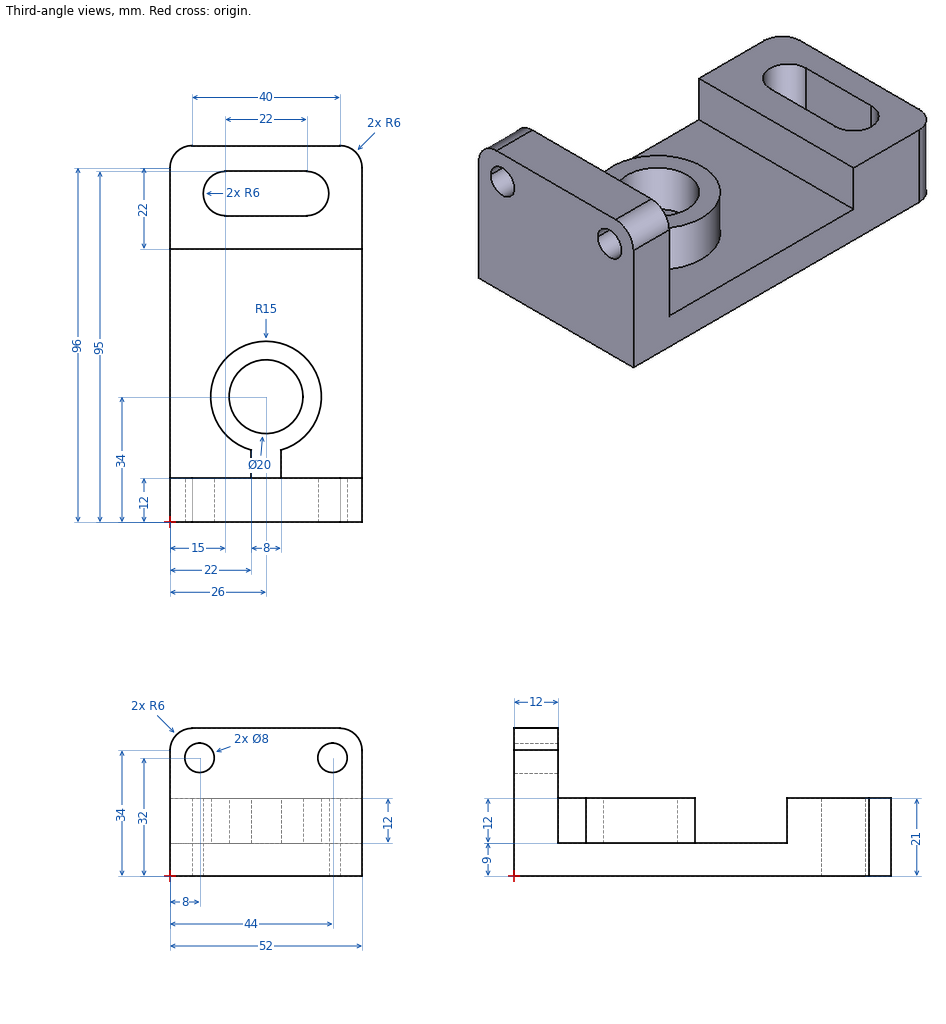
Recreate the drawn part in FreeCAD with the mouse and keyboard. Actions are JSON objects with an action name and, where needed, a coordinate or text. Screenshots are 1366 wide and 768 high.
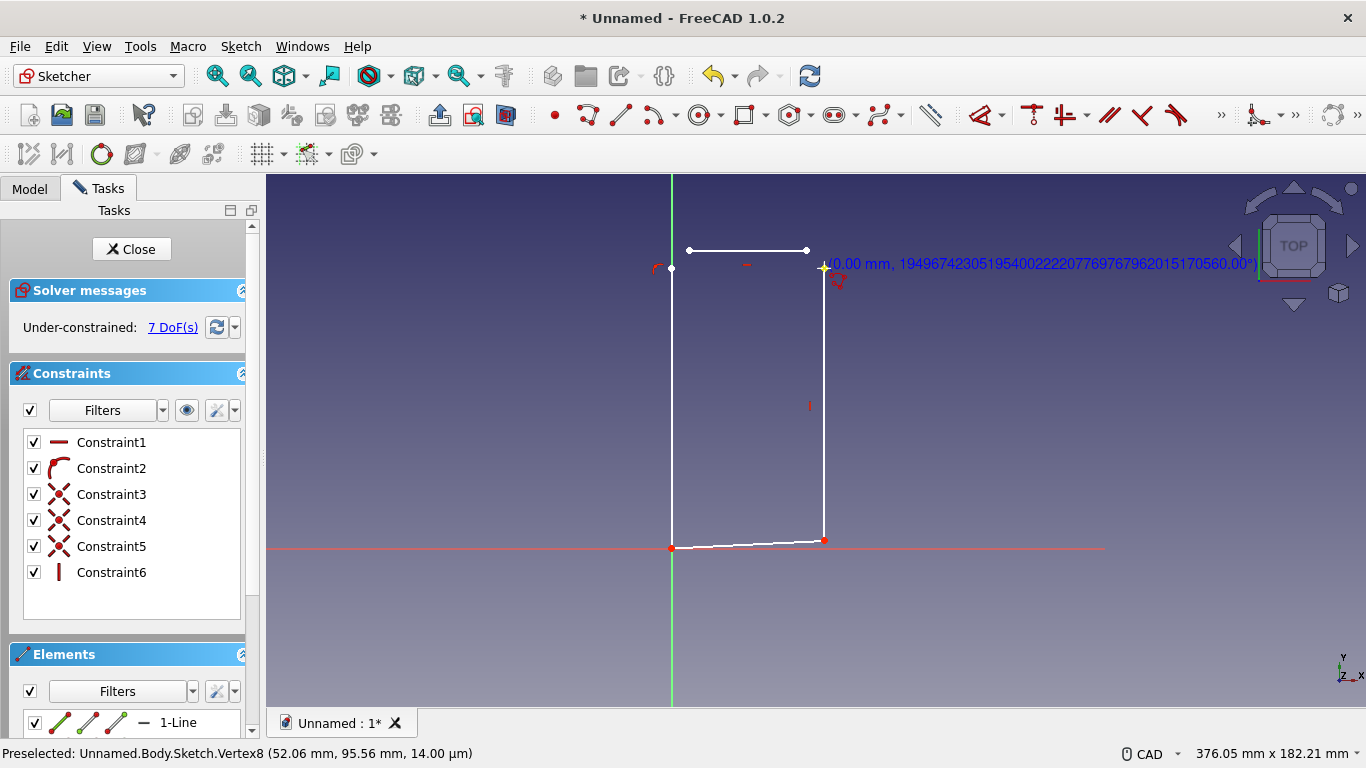
{"action": "left_click", "coordinate": [676, 116]}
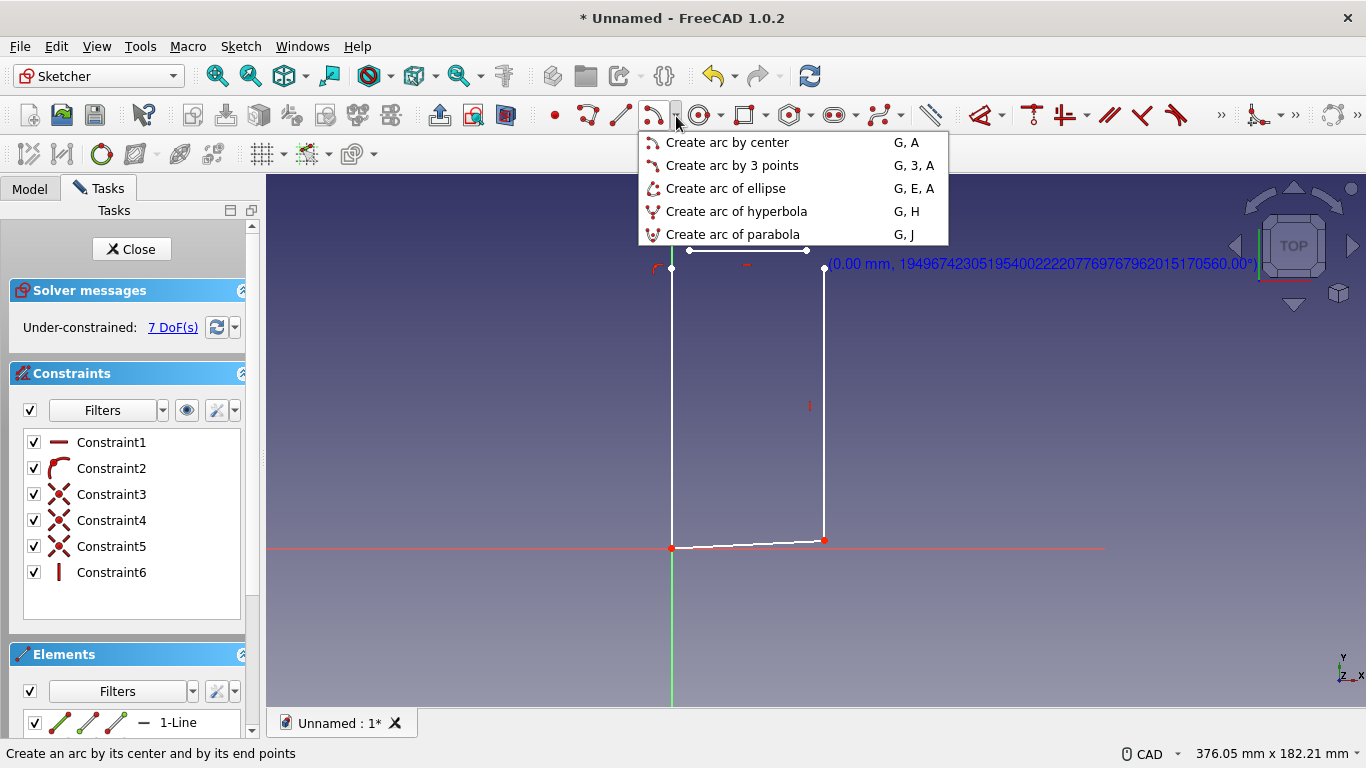
{"action": "left_click", "coordinate": [794, 166]}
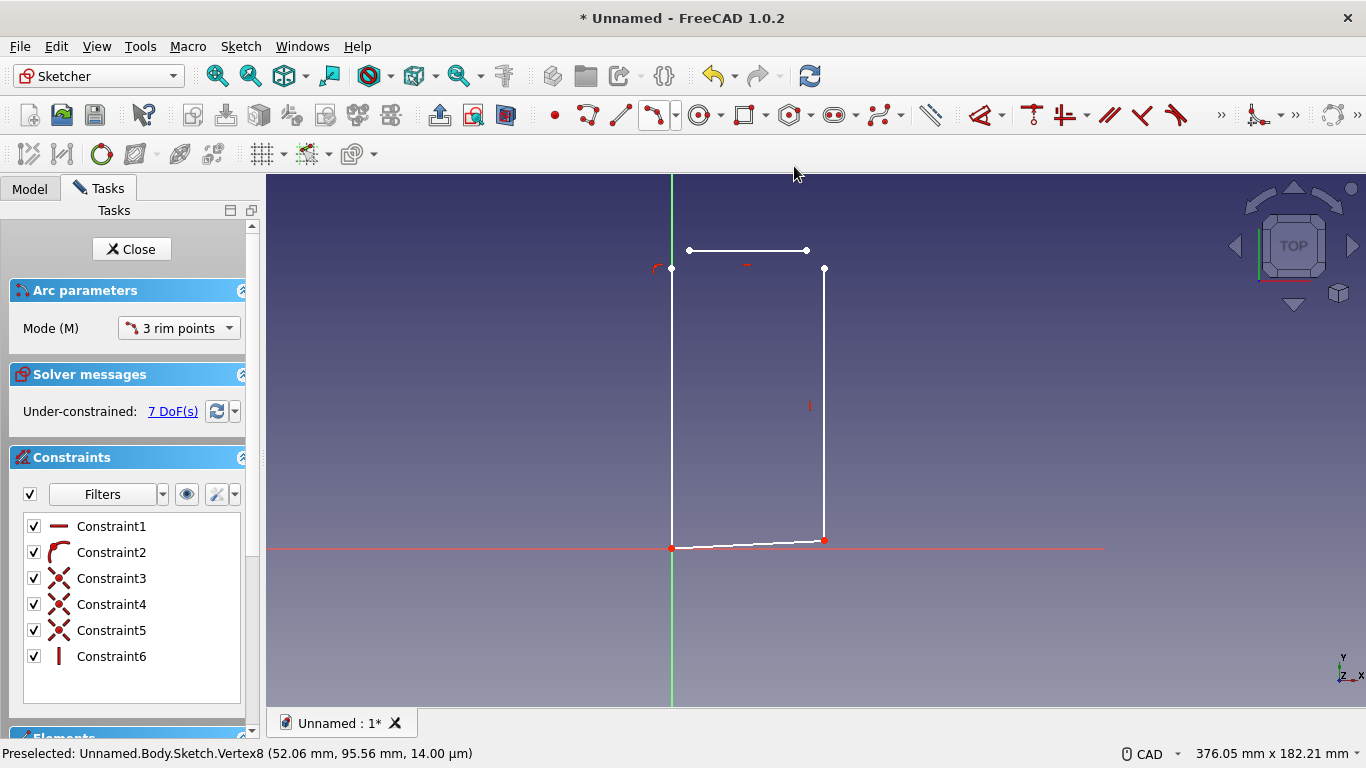
{"action": "left_click", "coordinate": [689, 251]}
{"action": "left_click", "coordinate": [672, 269]}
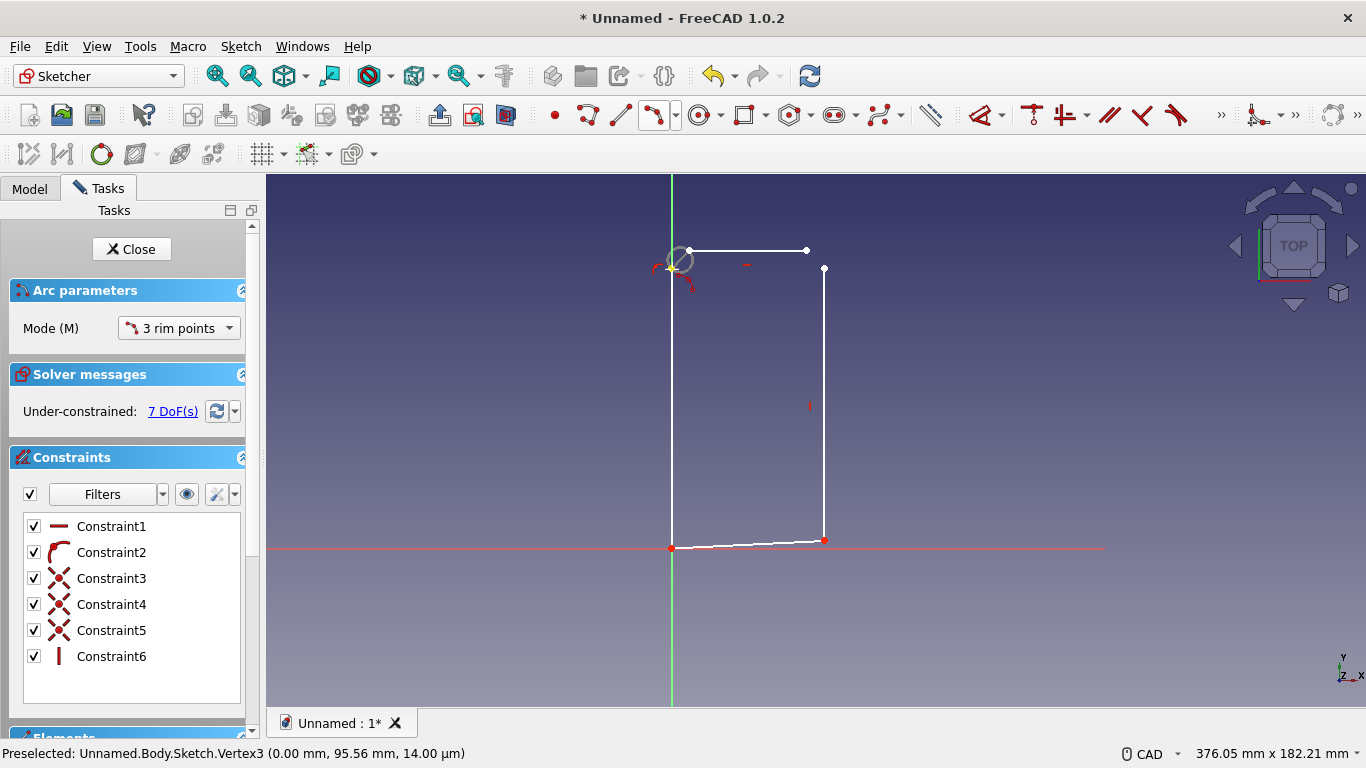
{"action": "scroll", "coordinate": [677, 255], "scroll_direction": "up", "scroll_amount": 6}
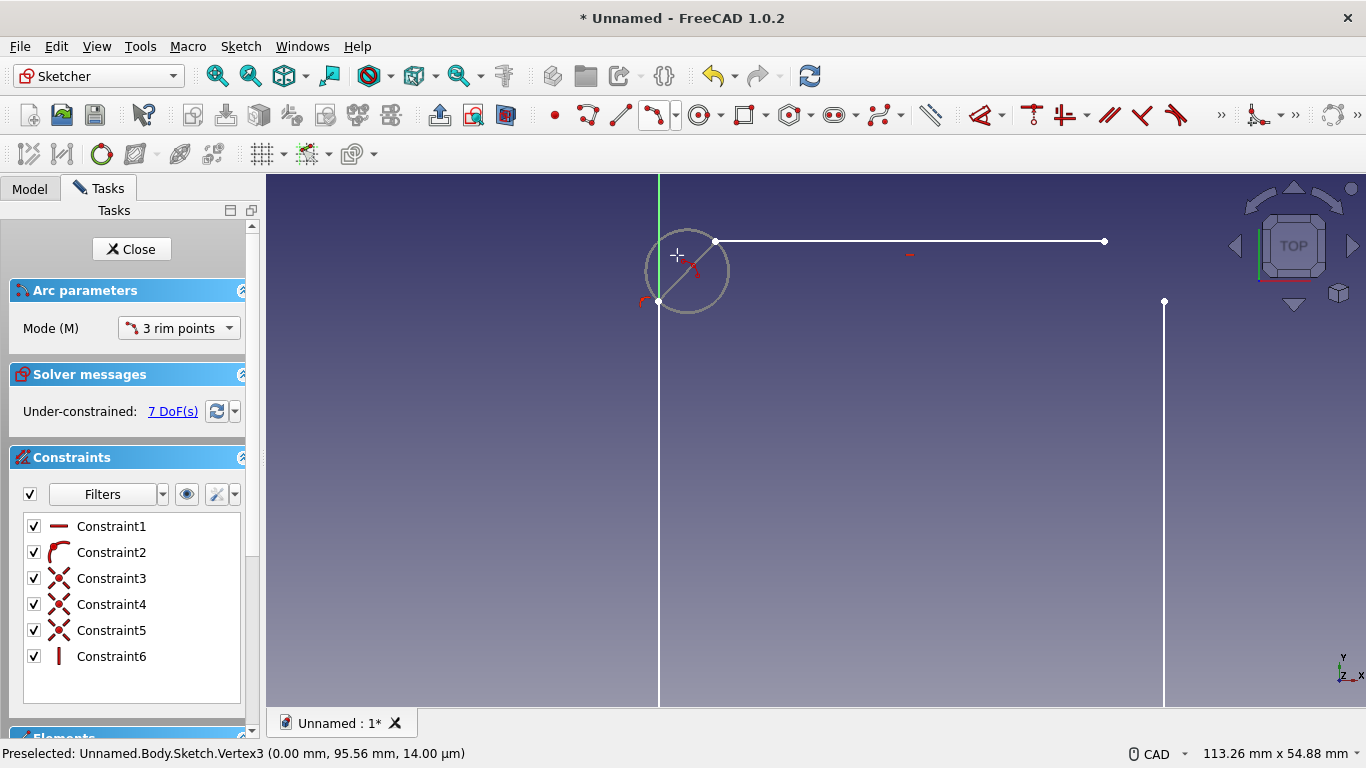
{"action": "left_click", "coordinate": [676, 256]}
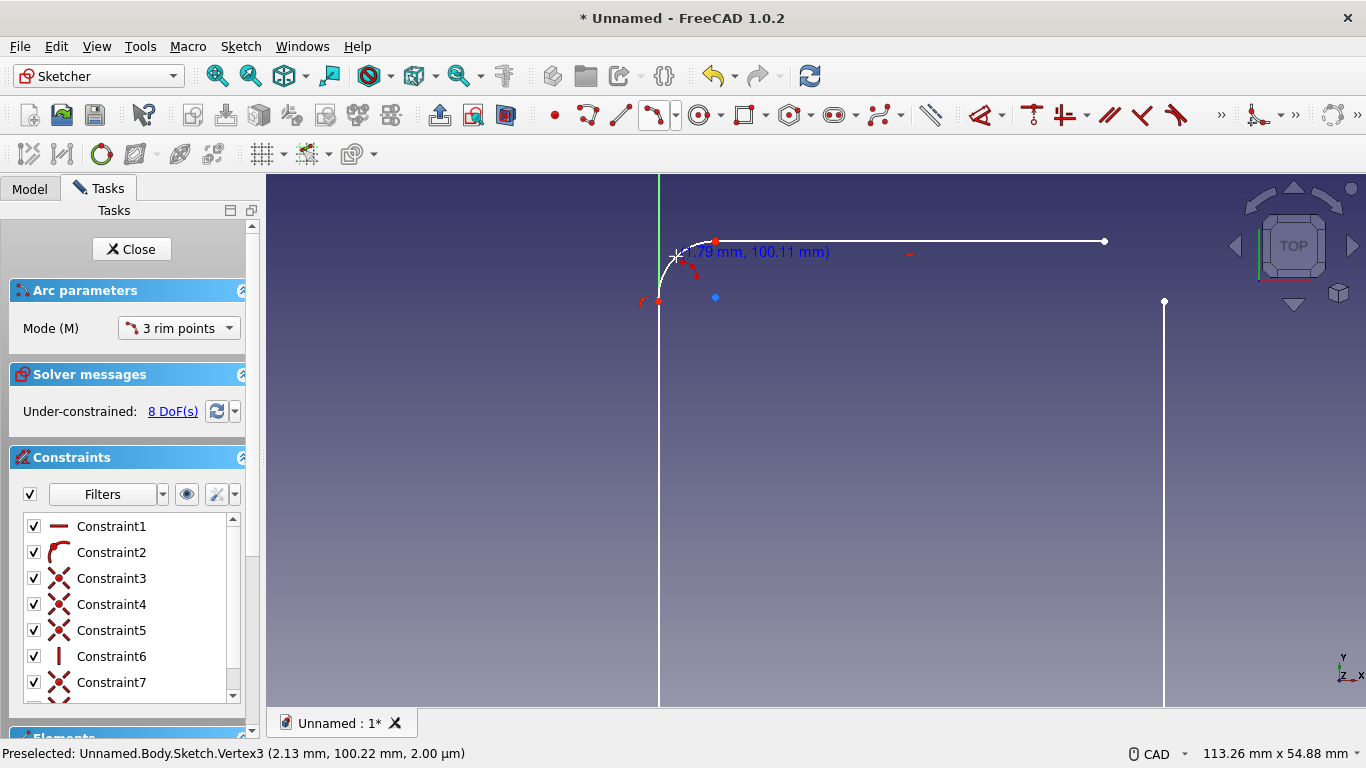
{"action": "left_click", "coordinate": [1164, 301]}
{"action": "left_click", "coordinate": [1104, 241]}
{"action": "left_click", "coordinate": [1147, 256]}
{"action": "key", "text": "Escape"}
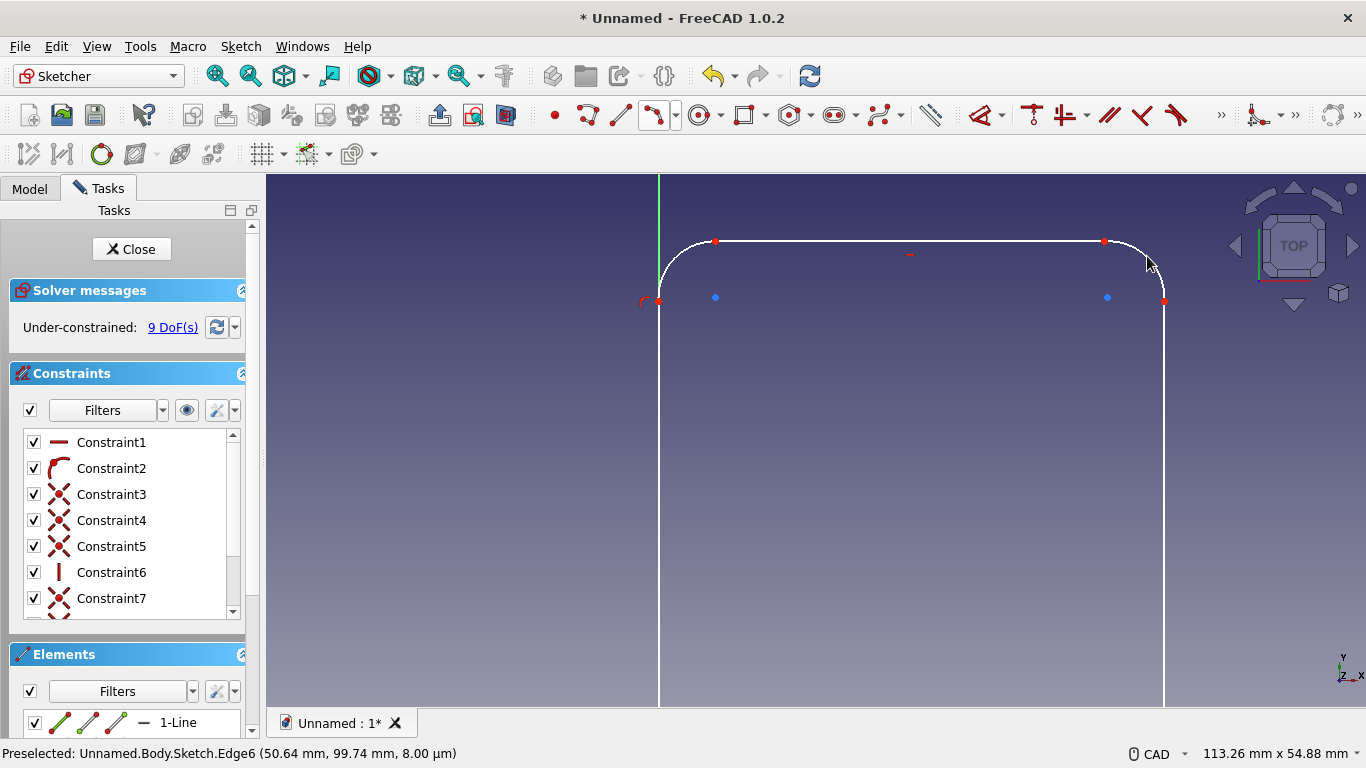
{"action": "left_click", "coordinate": [988, 241]}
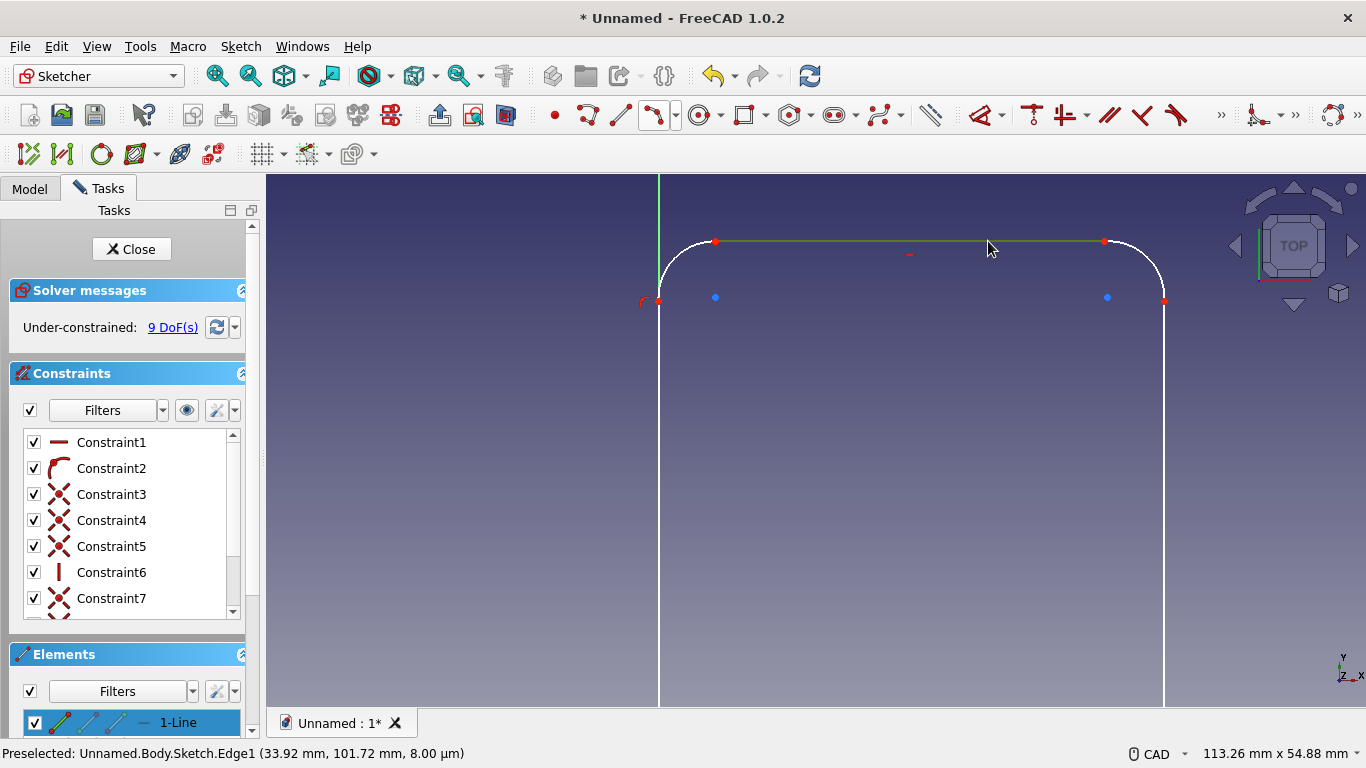
{"action": "left_click", "coordinate": [689, 248]}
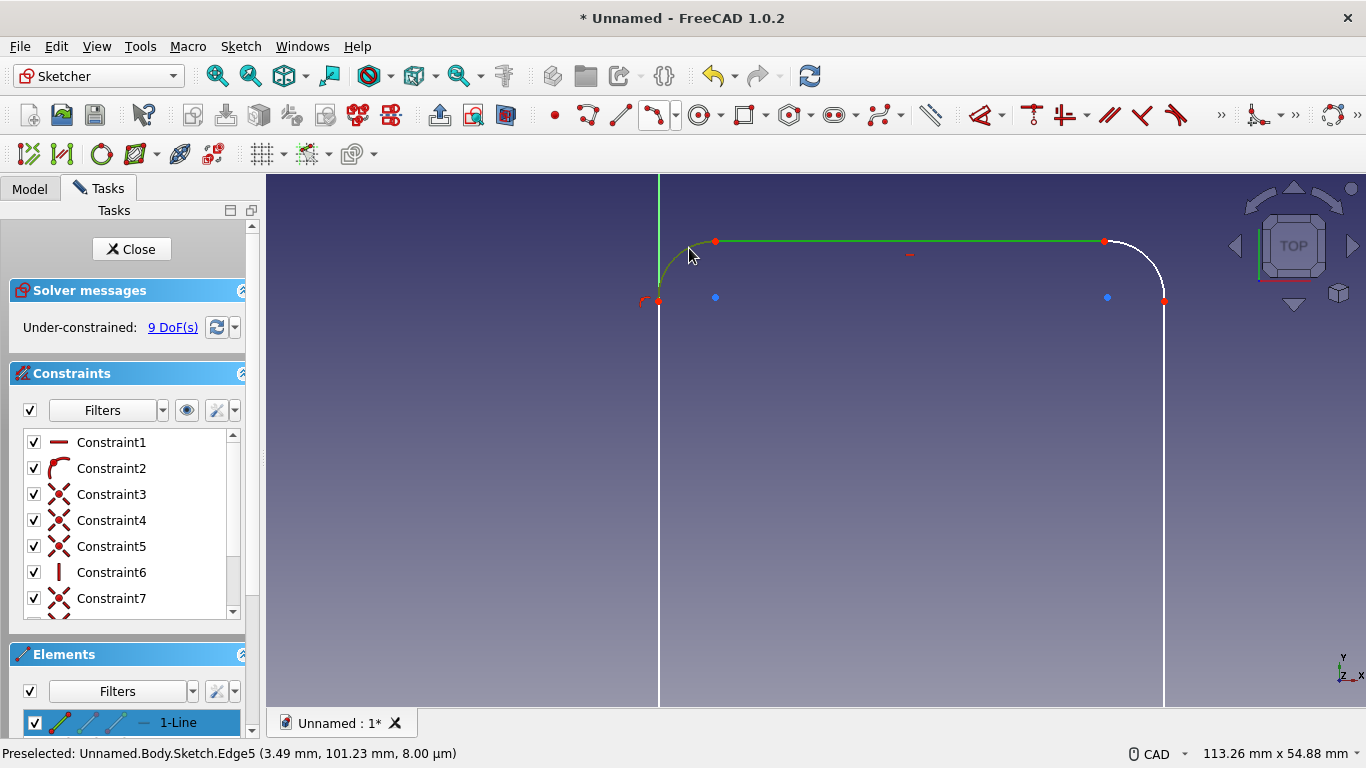
{"action": "left_click", "coordinate": [1176, 116]}